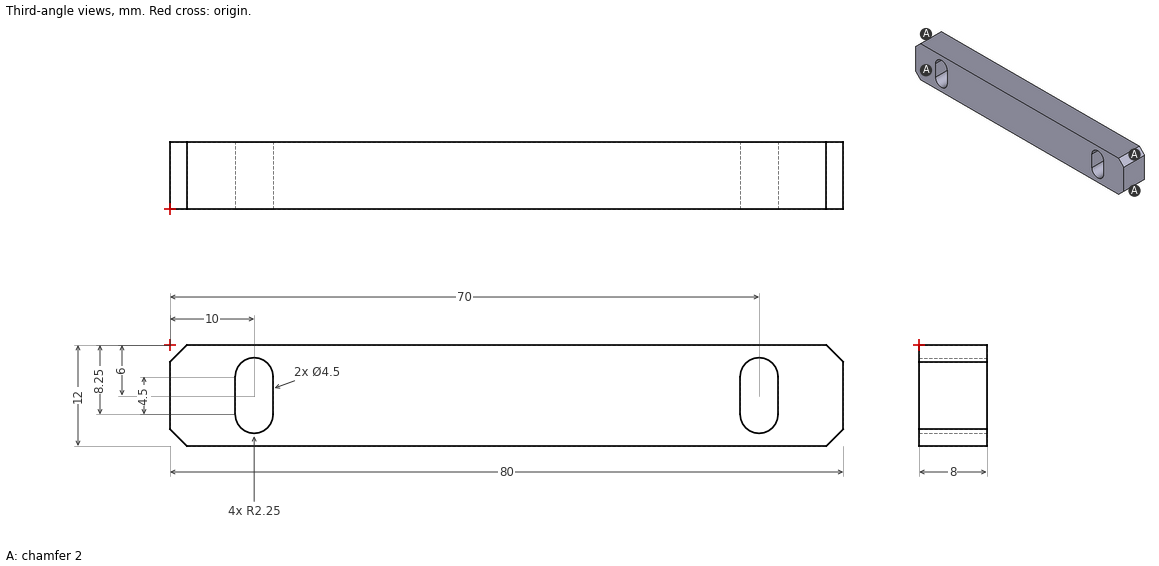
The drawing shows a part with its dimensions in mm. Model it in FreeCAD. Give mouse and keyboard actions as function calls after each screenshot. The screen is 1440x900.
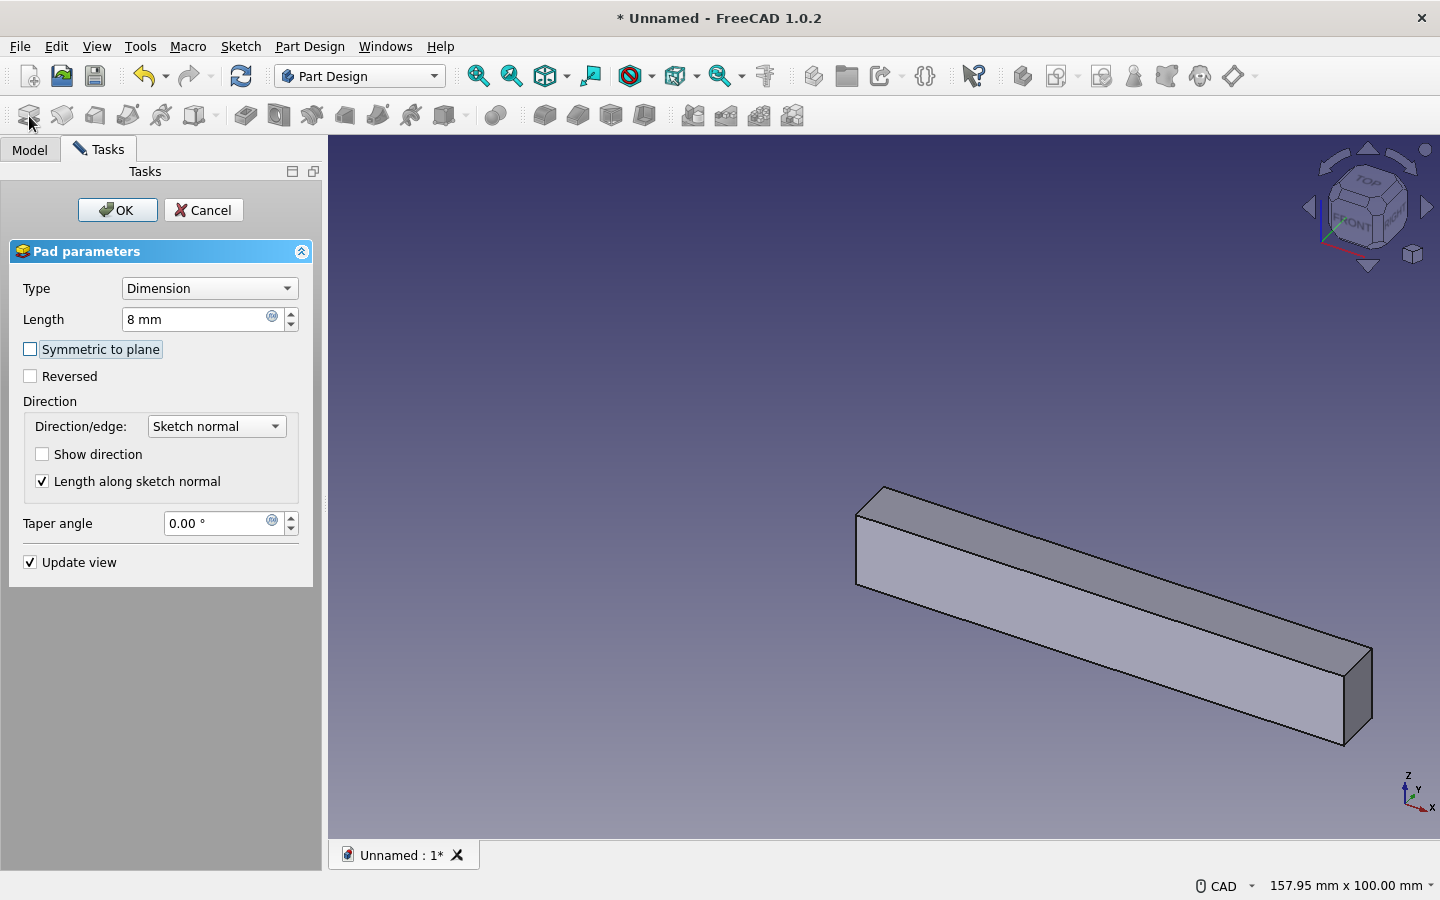
click(31, 376)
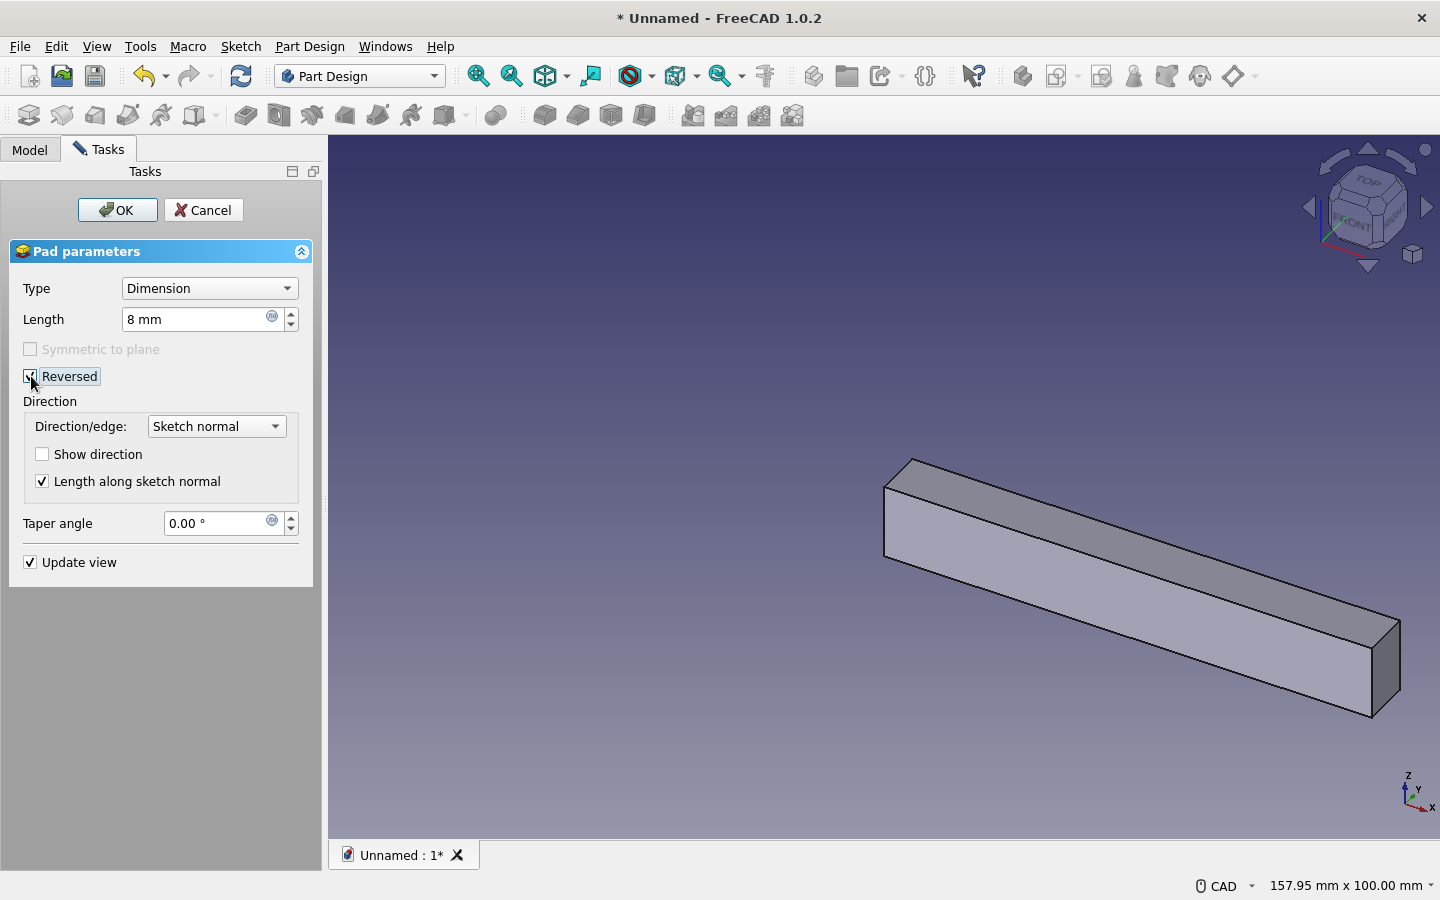
click(118, 210)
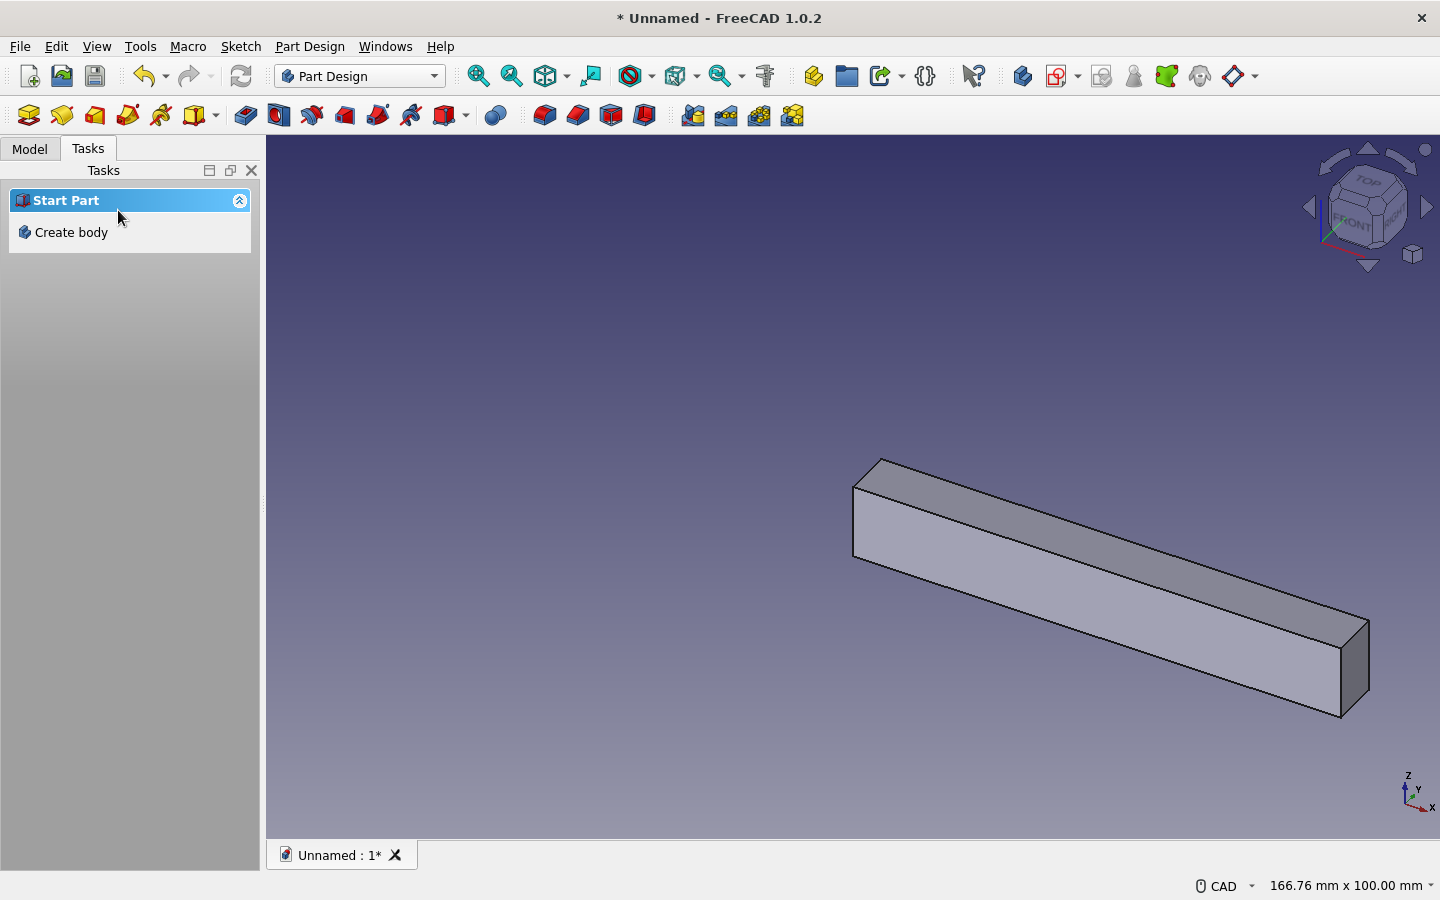
key(v)
key(f)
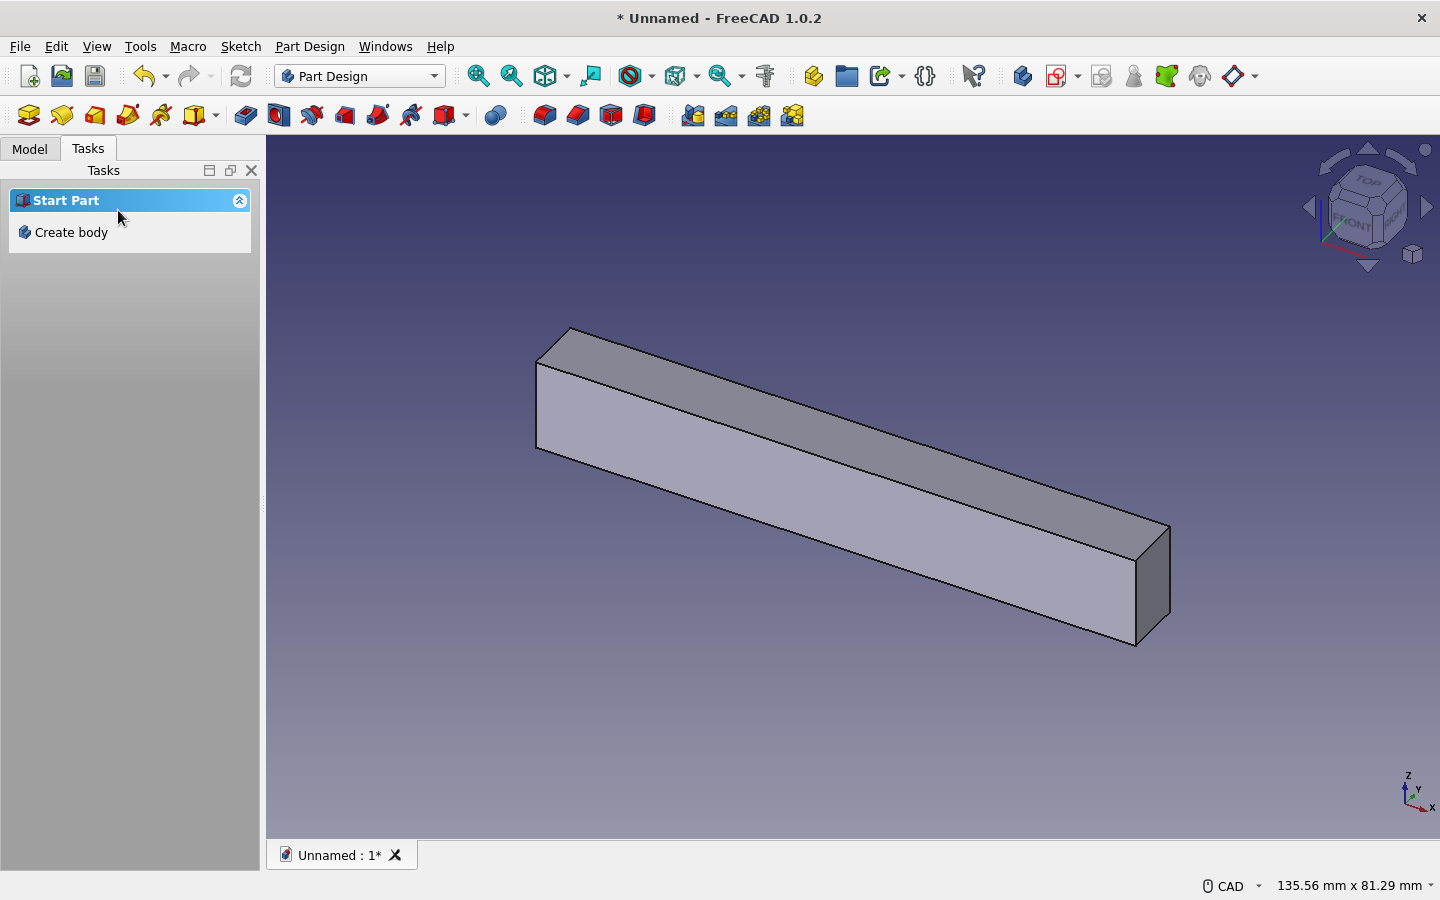
click(1153, 543)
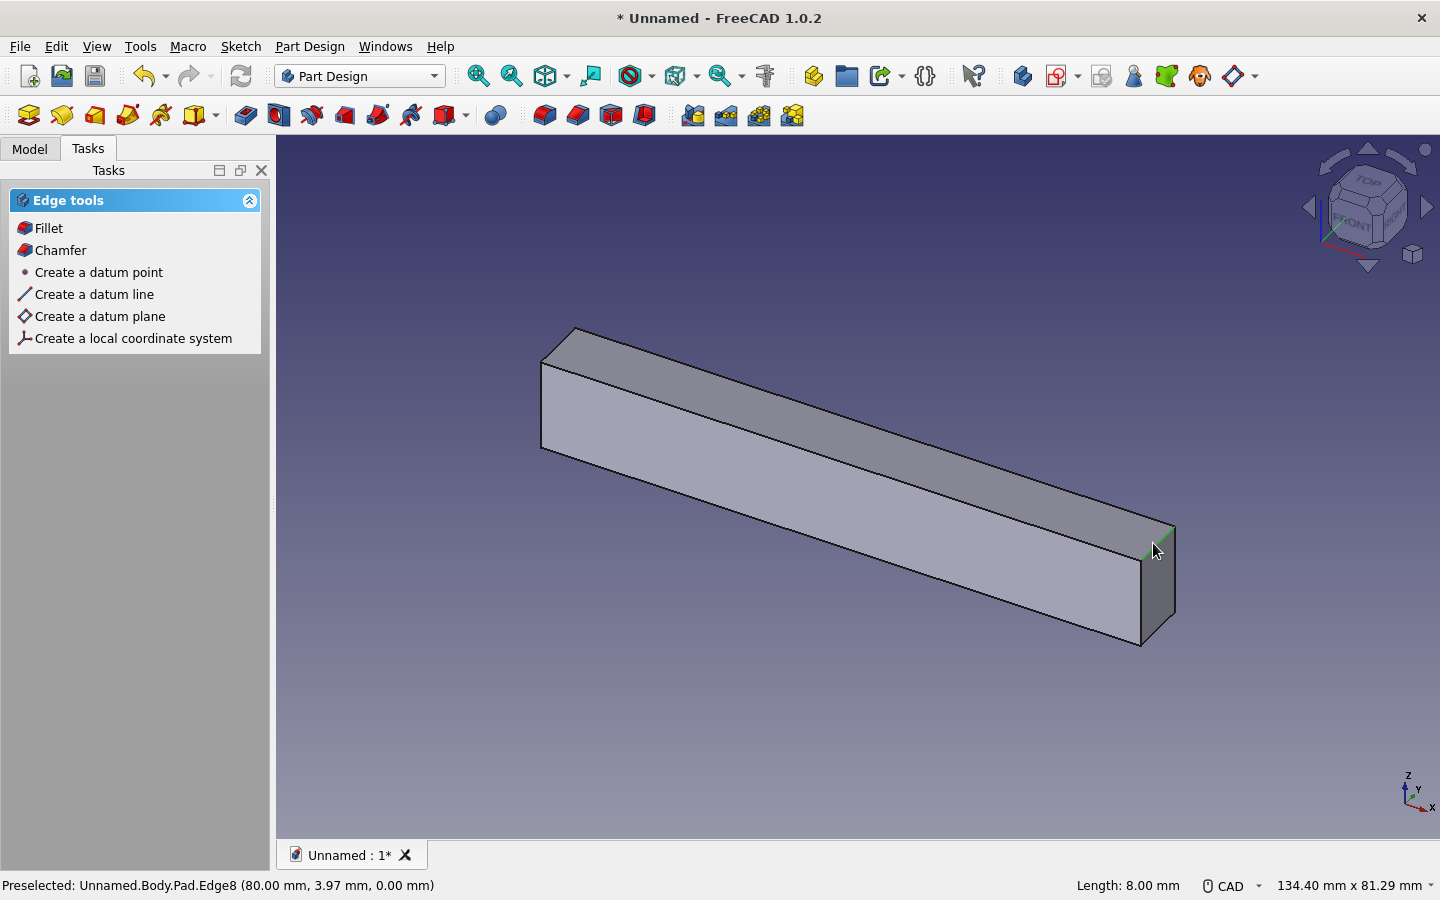
key(0)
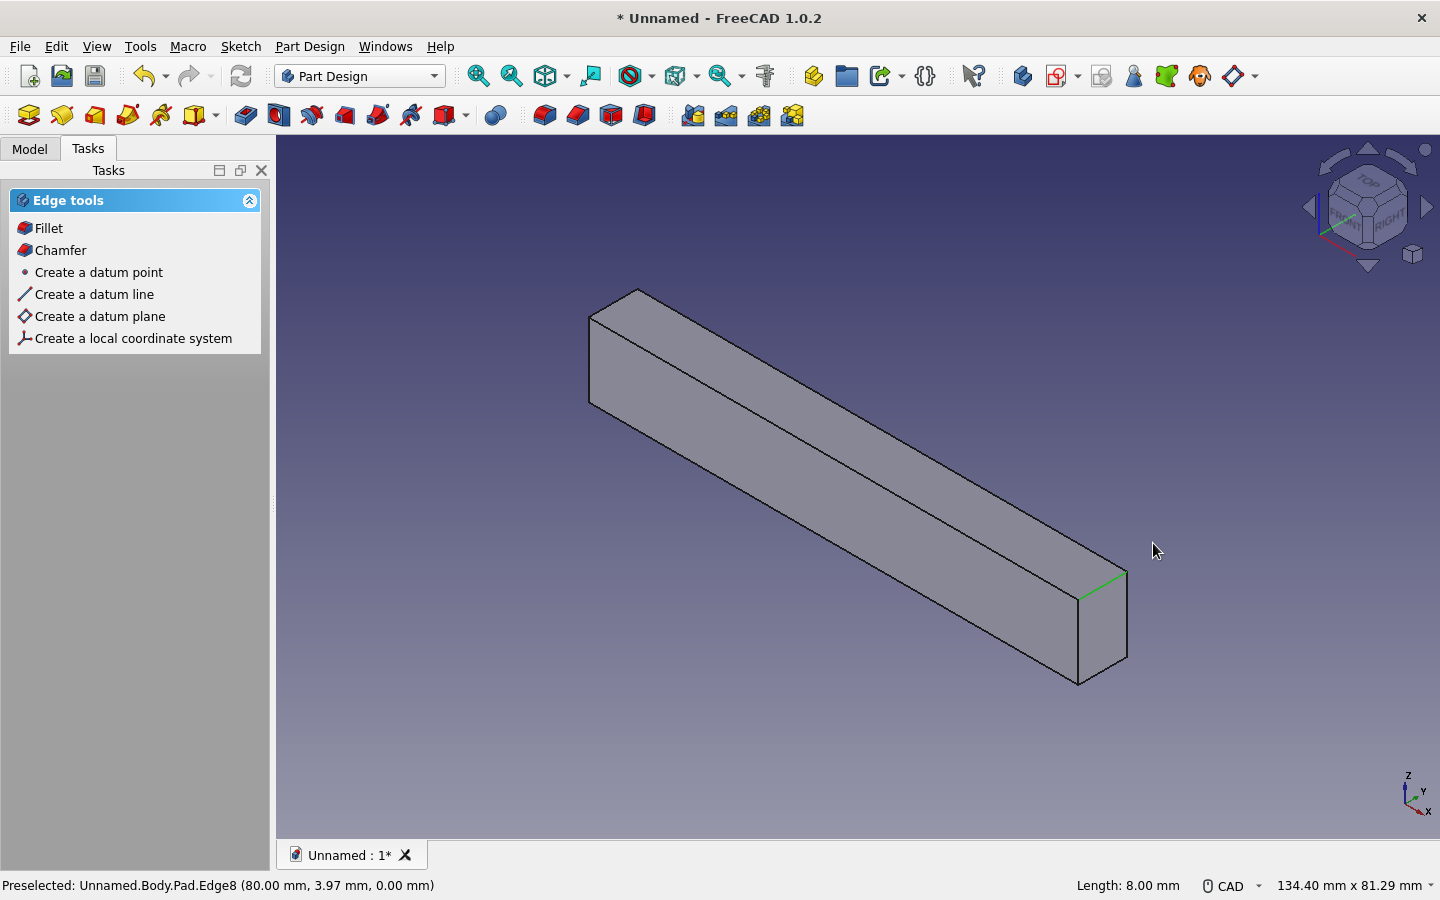
key(2)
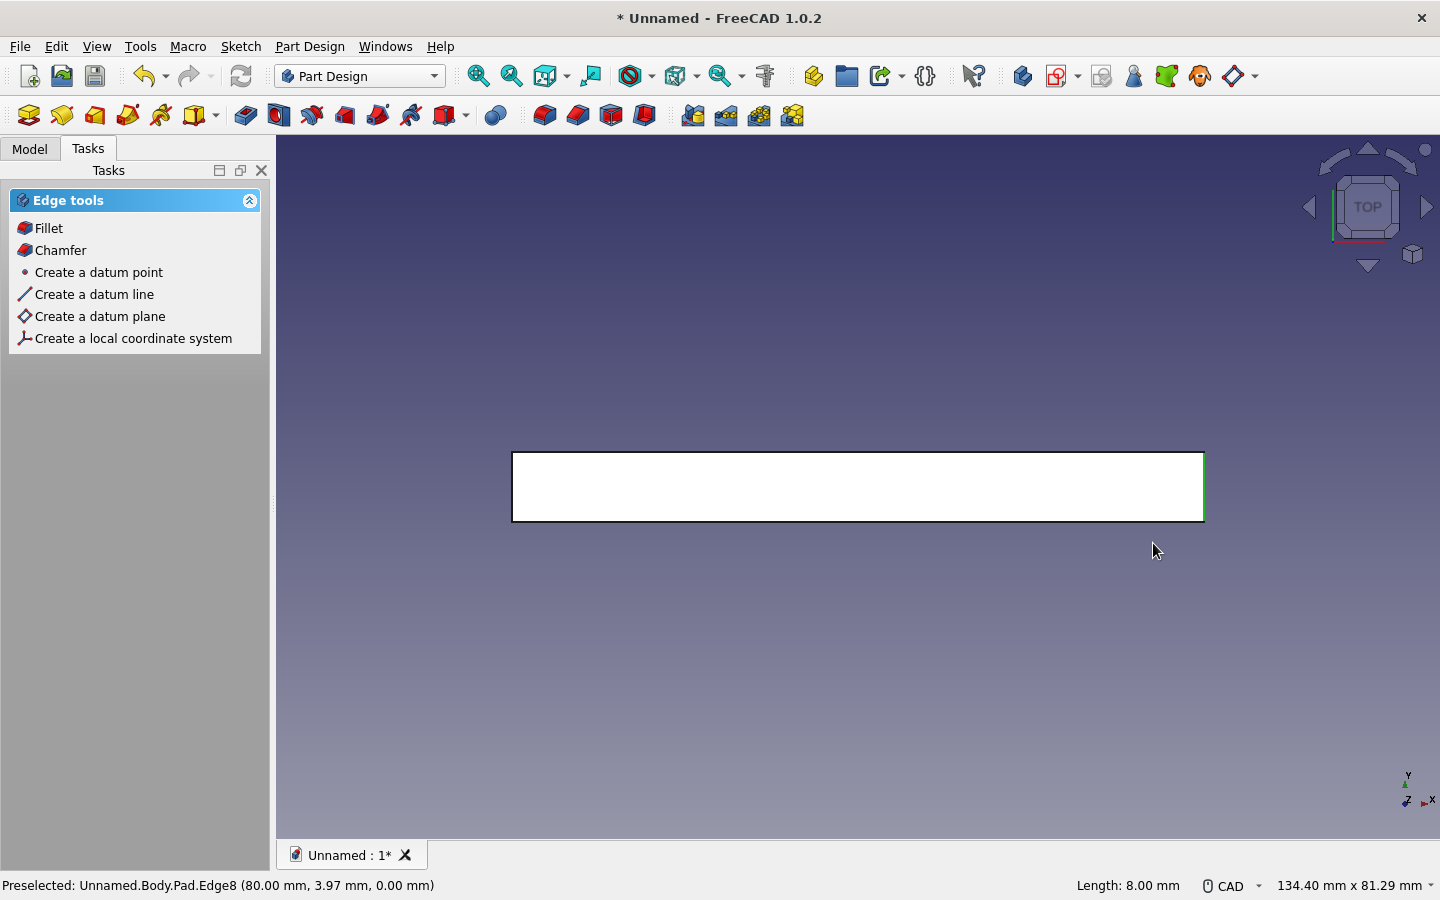
click(512, 486, ctrl)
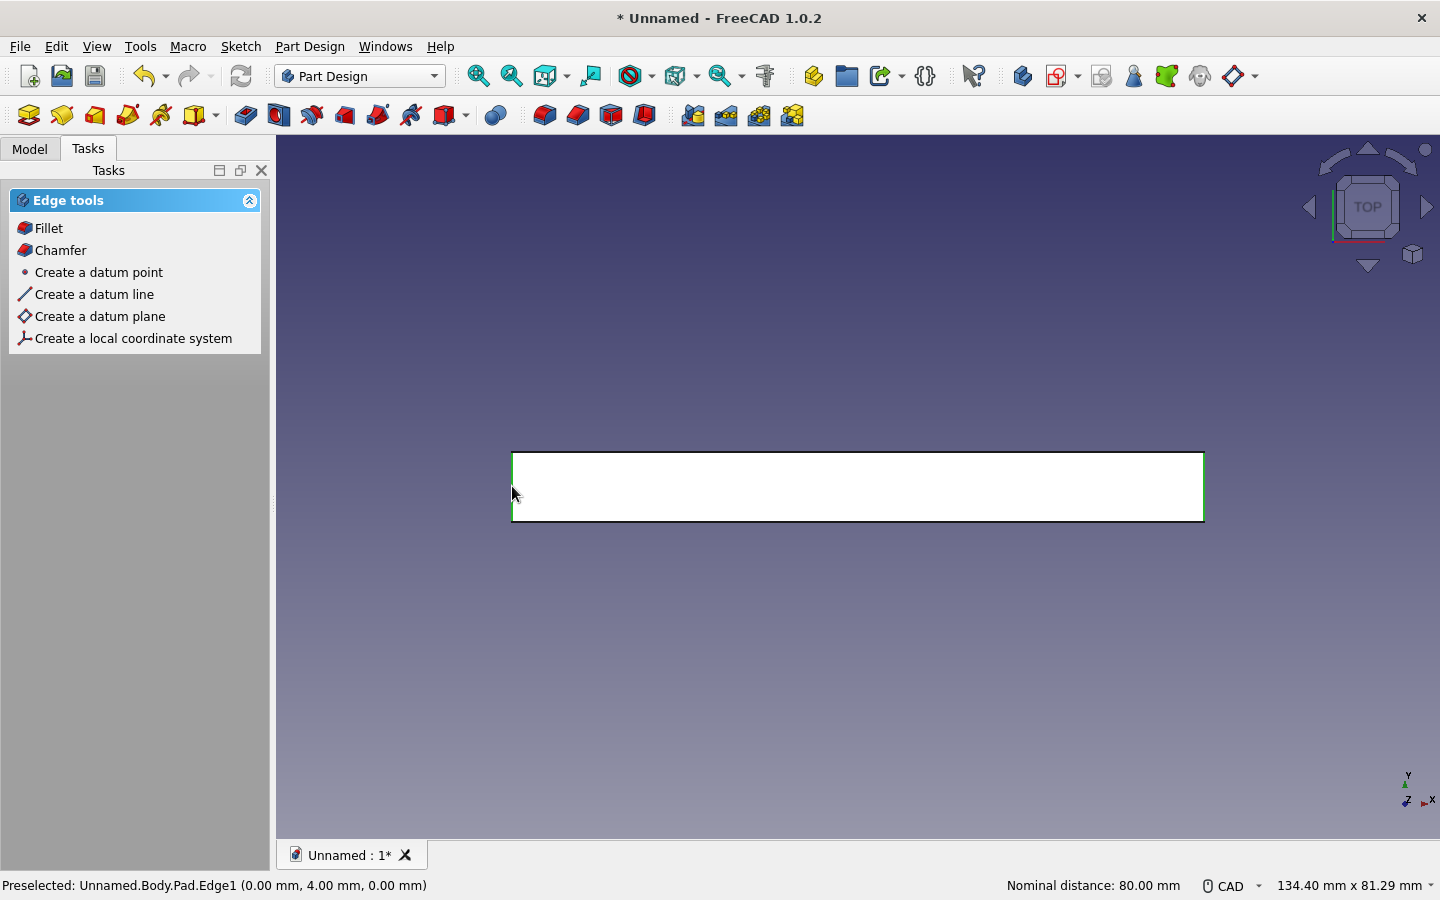
key(1)